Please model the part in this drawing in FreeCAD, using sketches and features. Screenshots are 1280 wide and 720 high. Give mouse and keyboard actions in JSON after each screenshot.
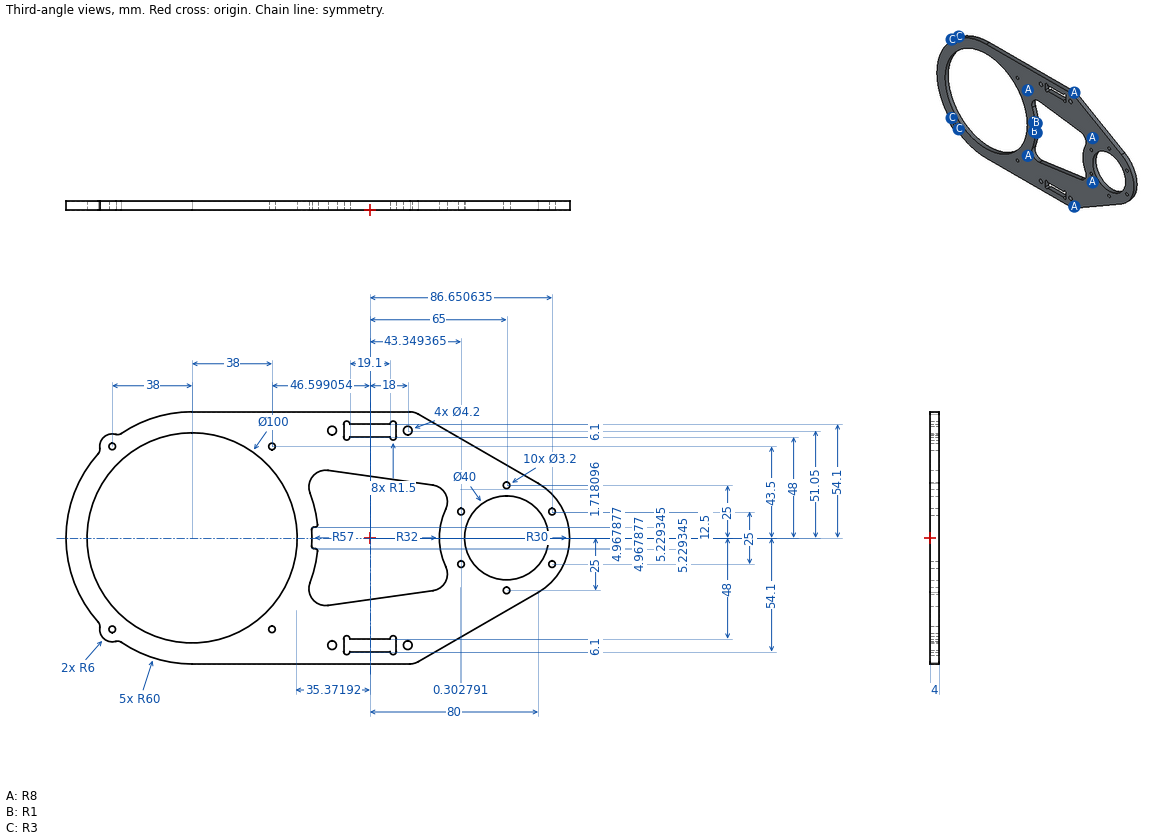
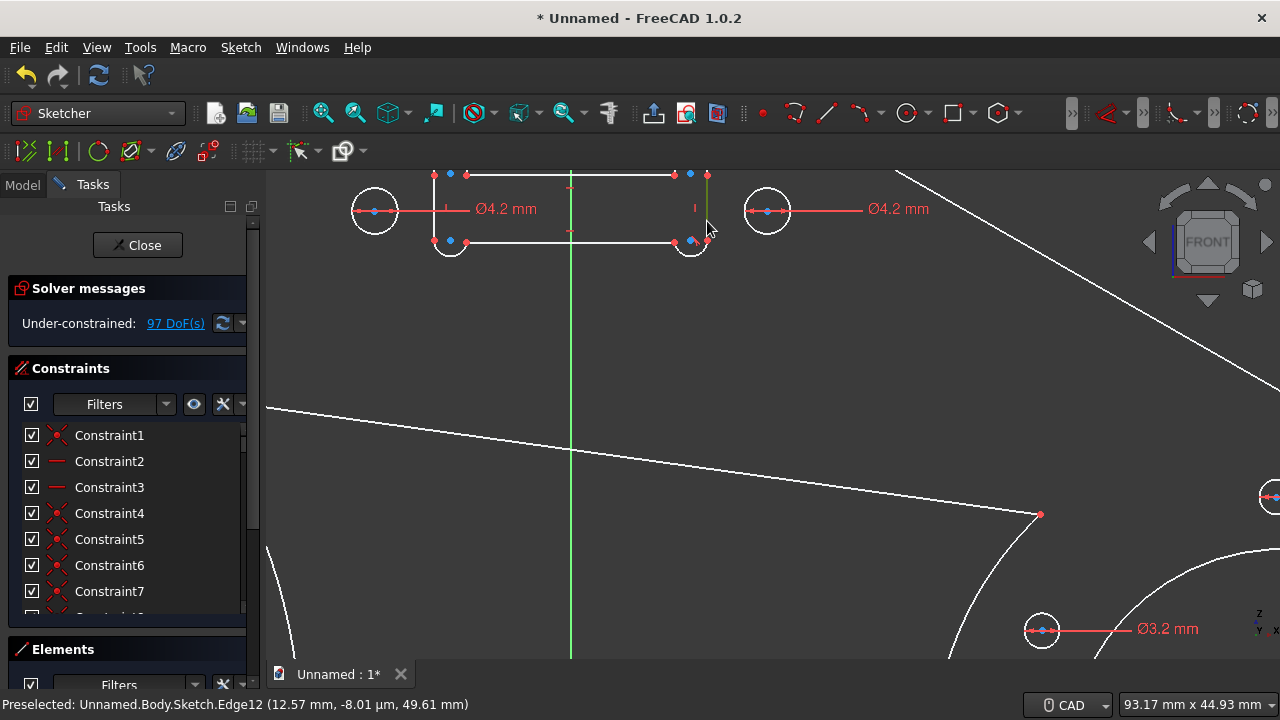
{"action": "scroll", "coordinate": [807, 327], "scroll_direction": "down", "scroll_amount": 8}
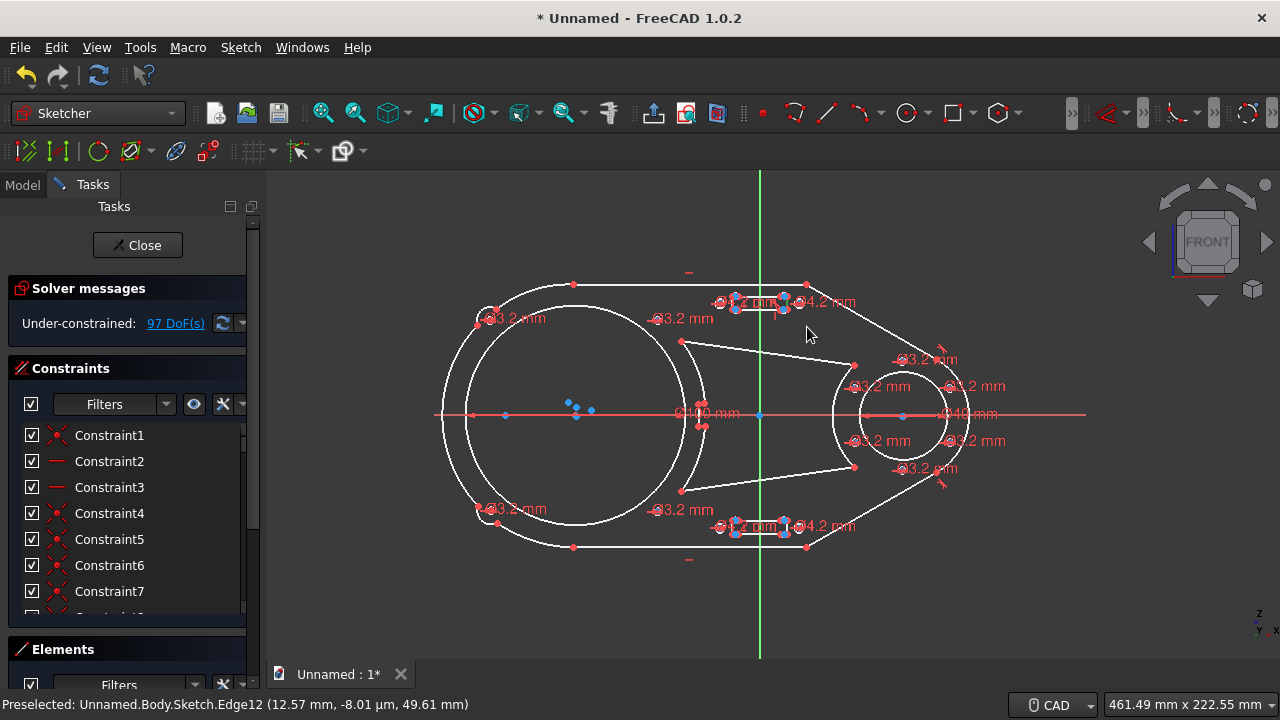
{"action": "scroll", "coordinate": [786, 294], "scroll_direction": "up", "scroll_amount": 8}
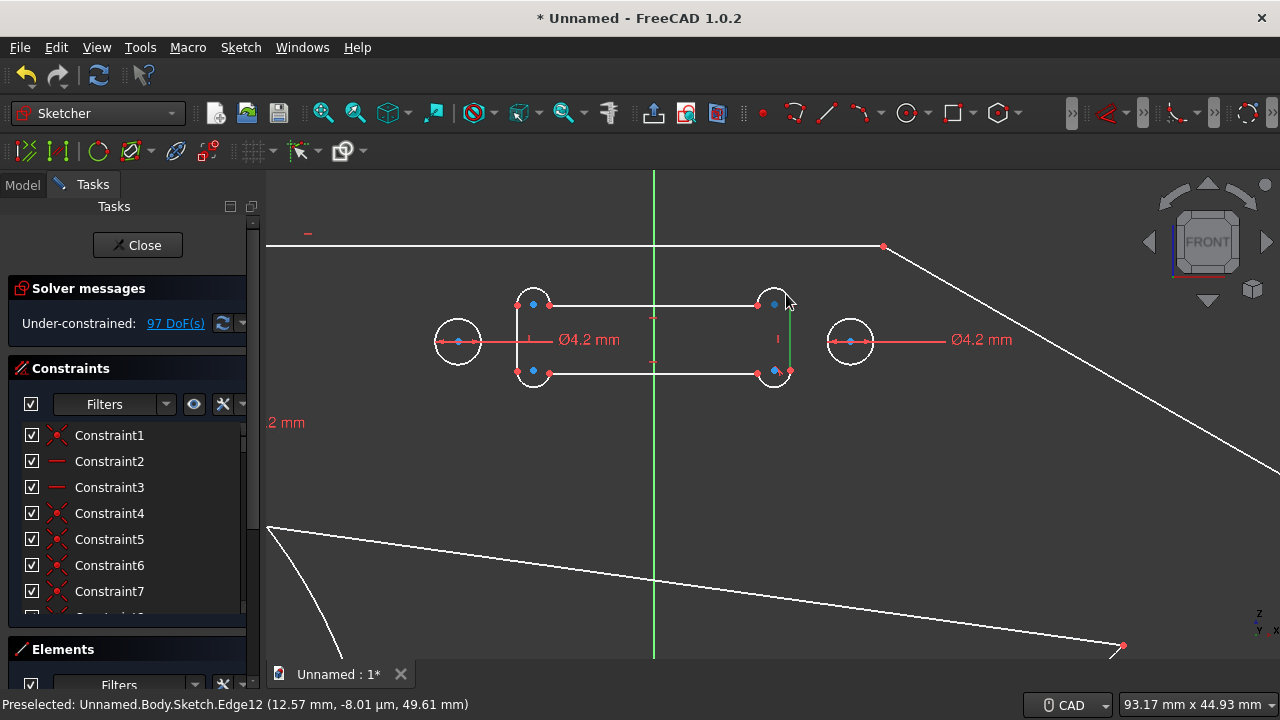
{"action": "left_click", "coordinate": [784, 292]}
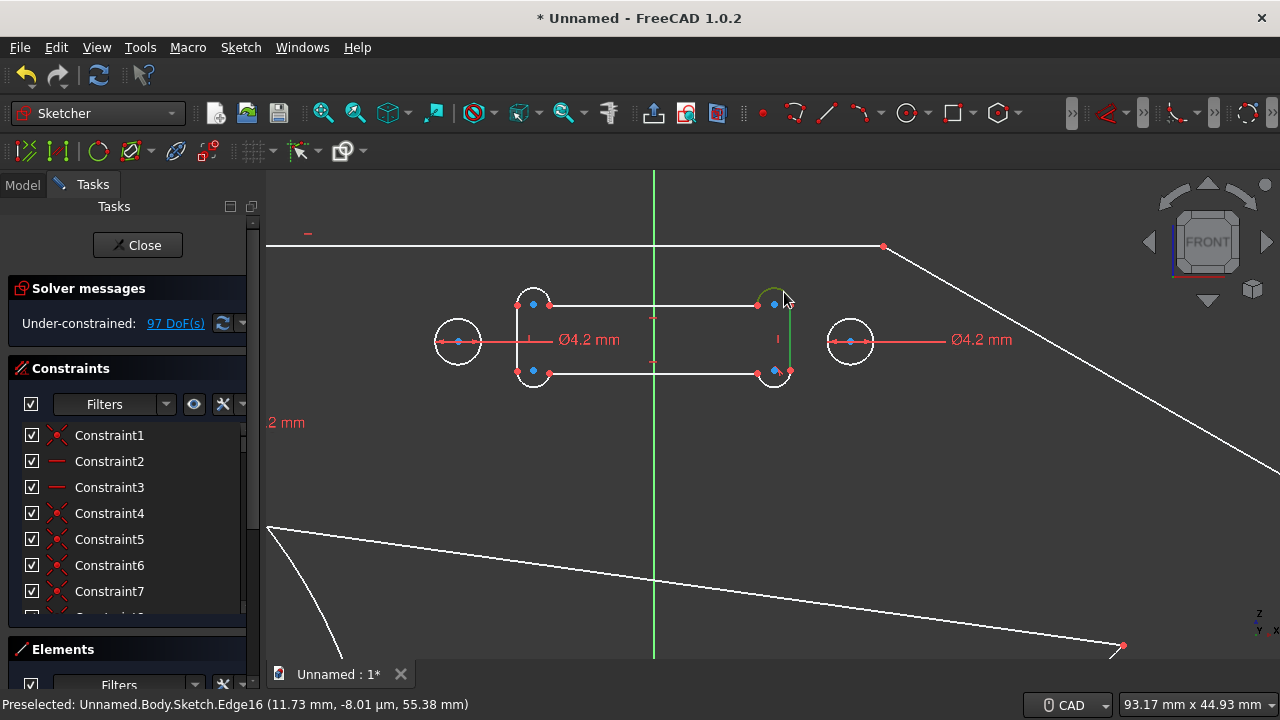
{"action": "key", "text": "t"}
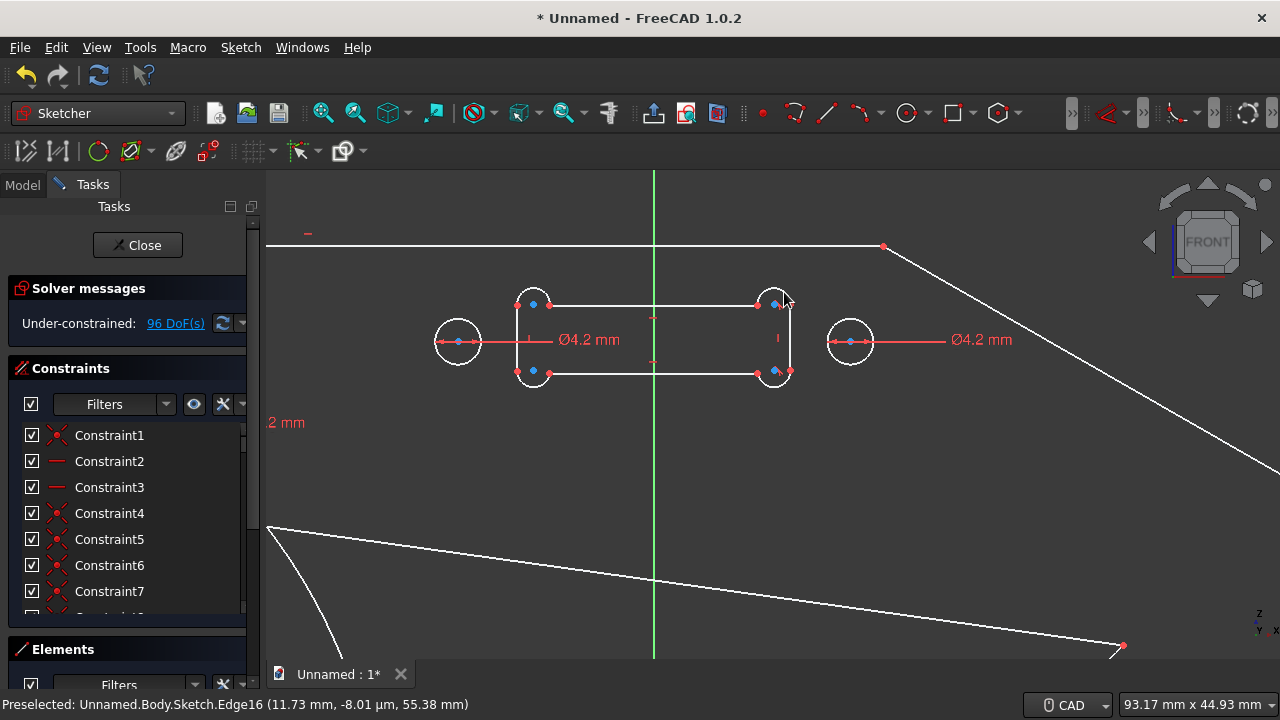
{"action": "left_click", "coordinate": [517, 325]}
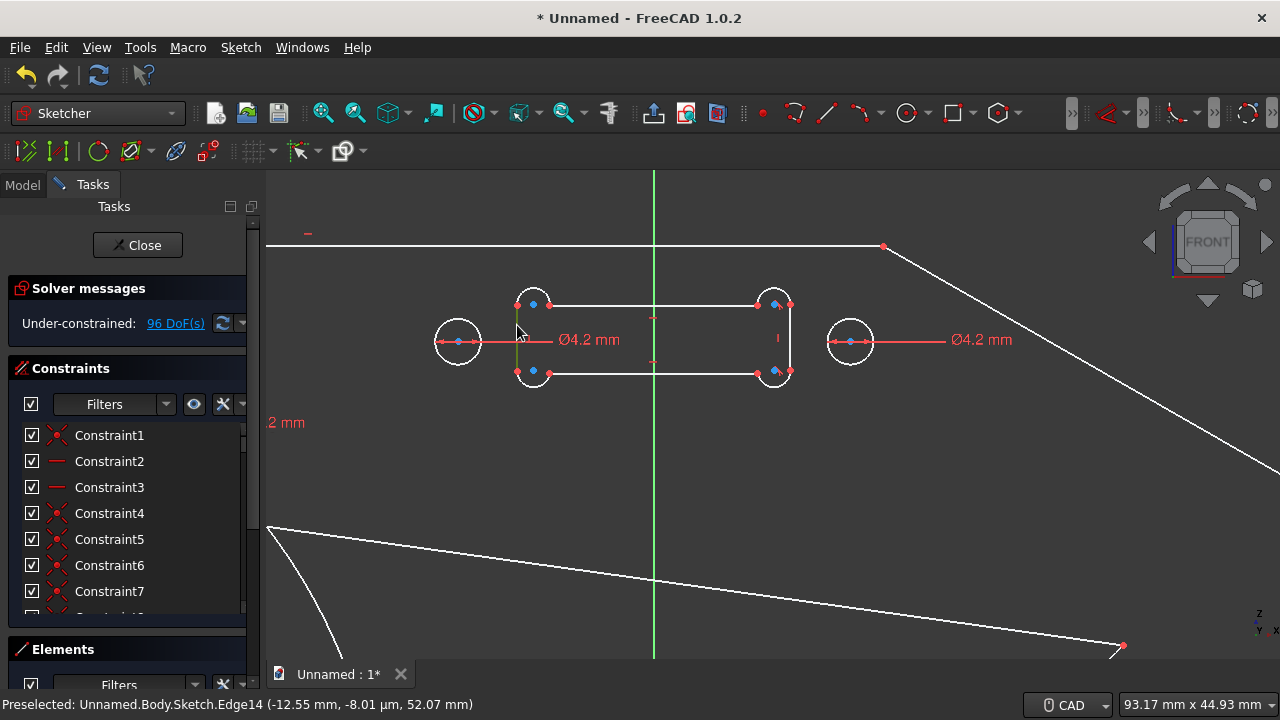
{"action": "left_click", "coordinate": [544, 292]}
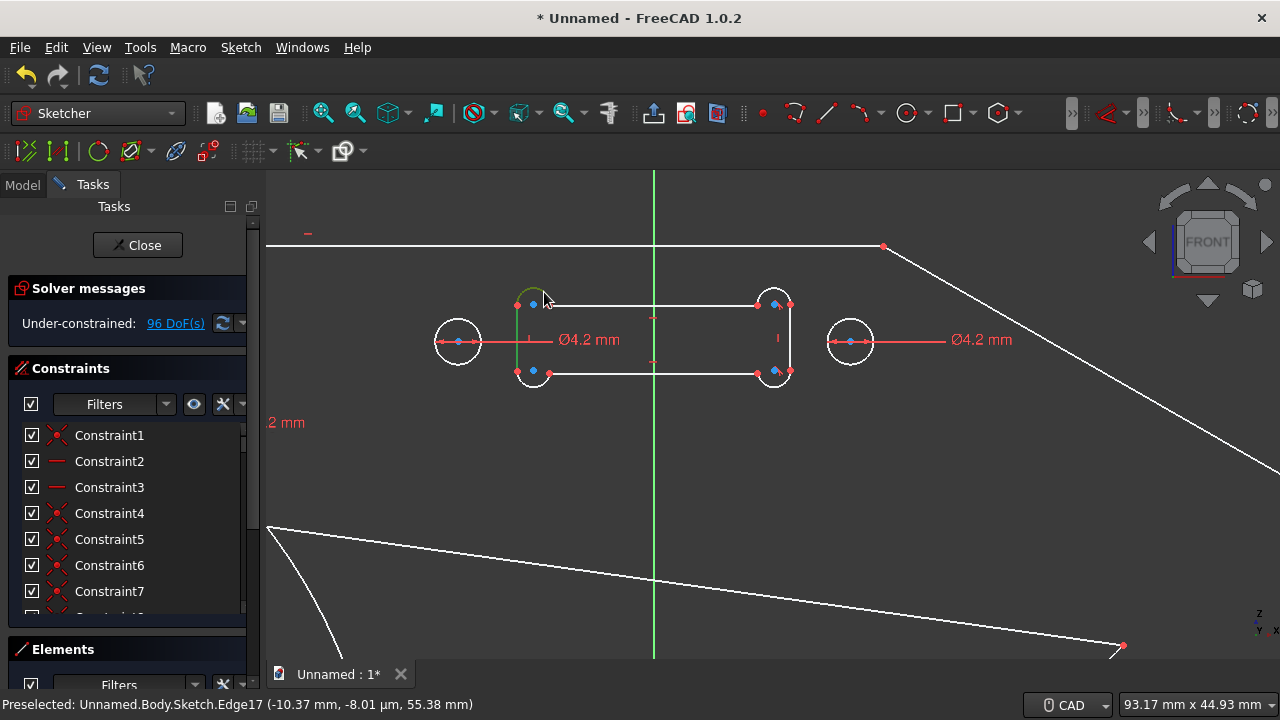
{"action": "key", "text": "t"}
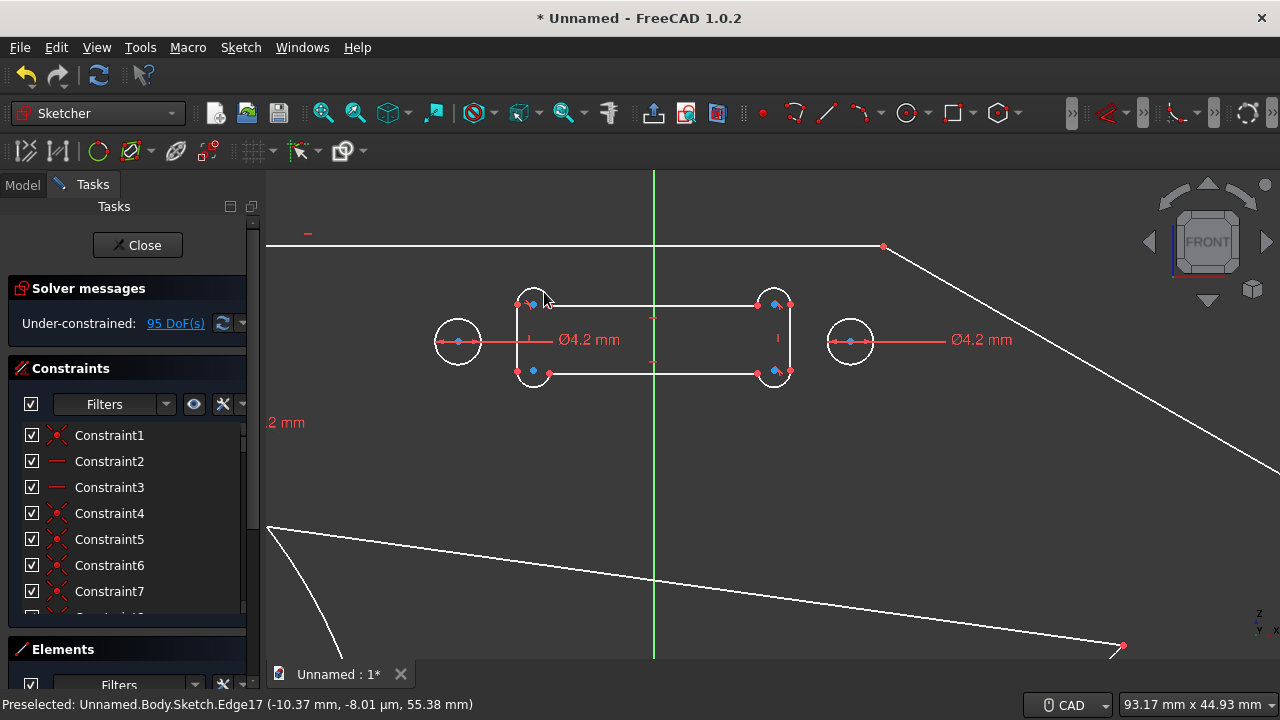
{"action": "left_click", "coordinate": [517, 325]}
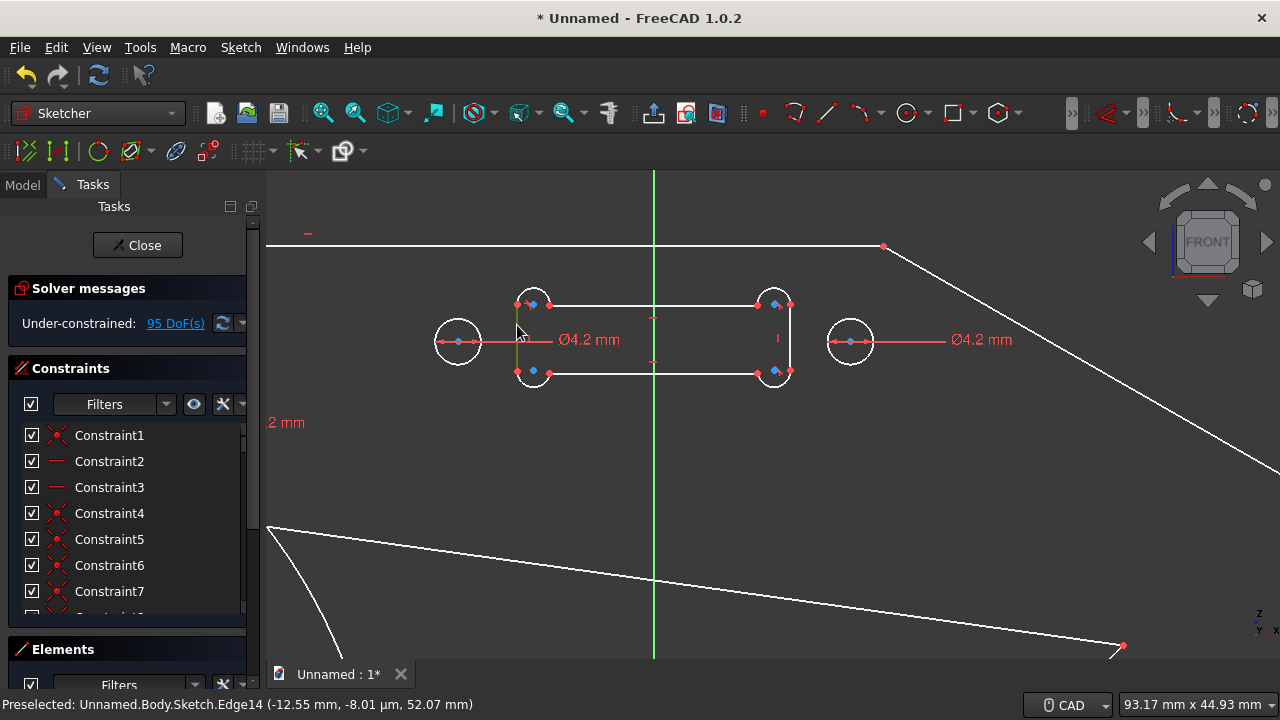
{"action": "left_click", "coordinate": [524, 384]}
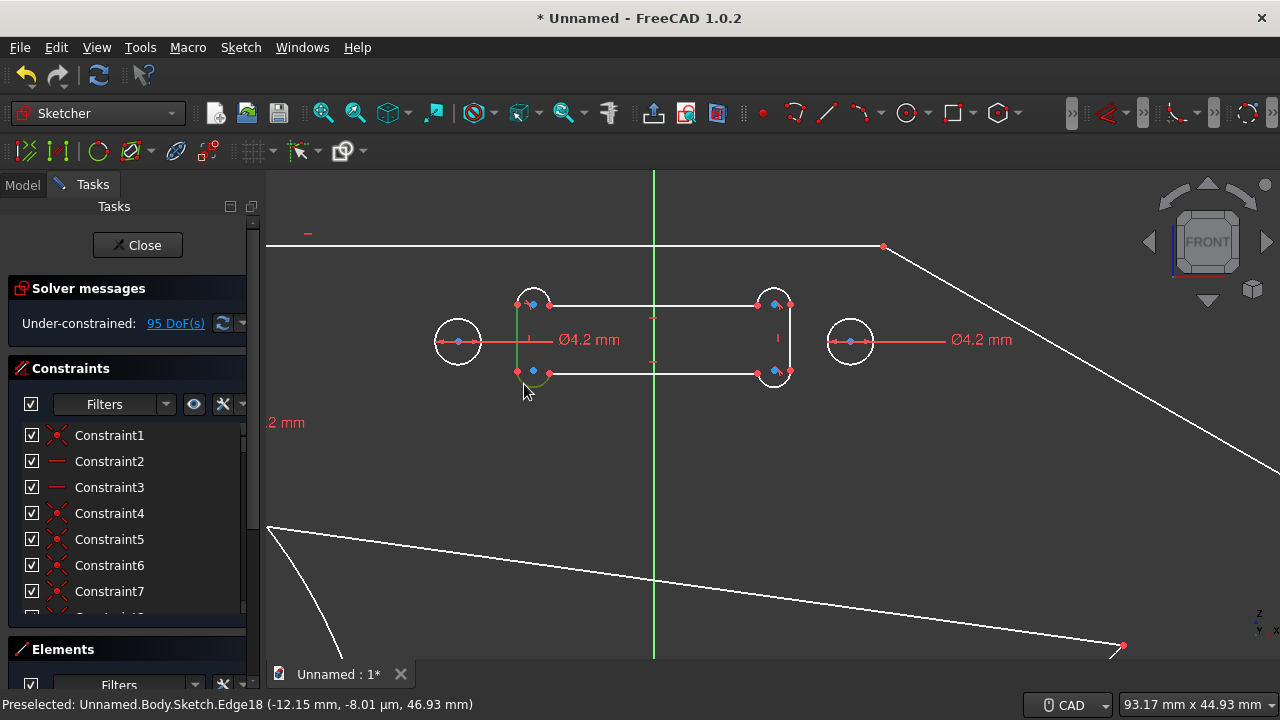
{"action": "key", "text": "t"}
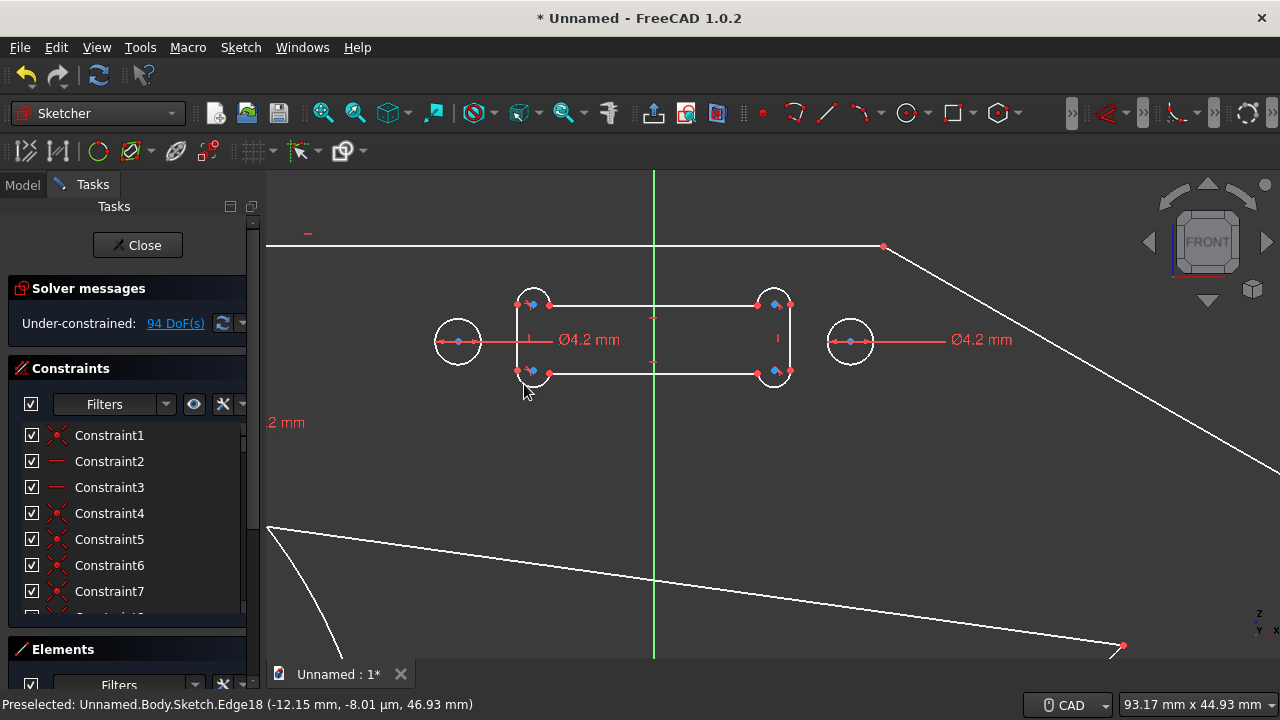
{"action": "scroll", "coordinate": [786, 294], "scroll_direction": "down", "scroll_amount": 8}